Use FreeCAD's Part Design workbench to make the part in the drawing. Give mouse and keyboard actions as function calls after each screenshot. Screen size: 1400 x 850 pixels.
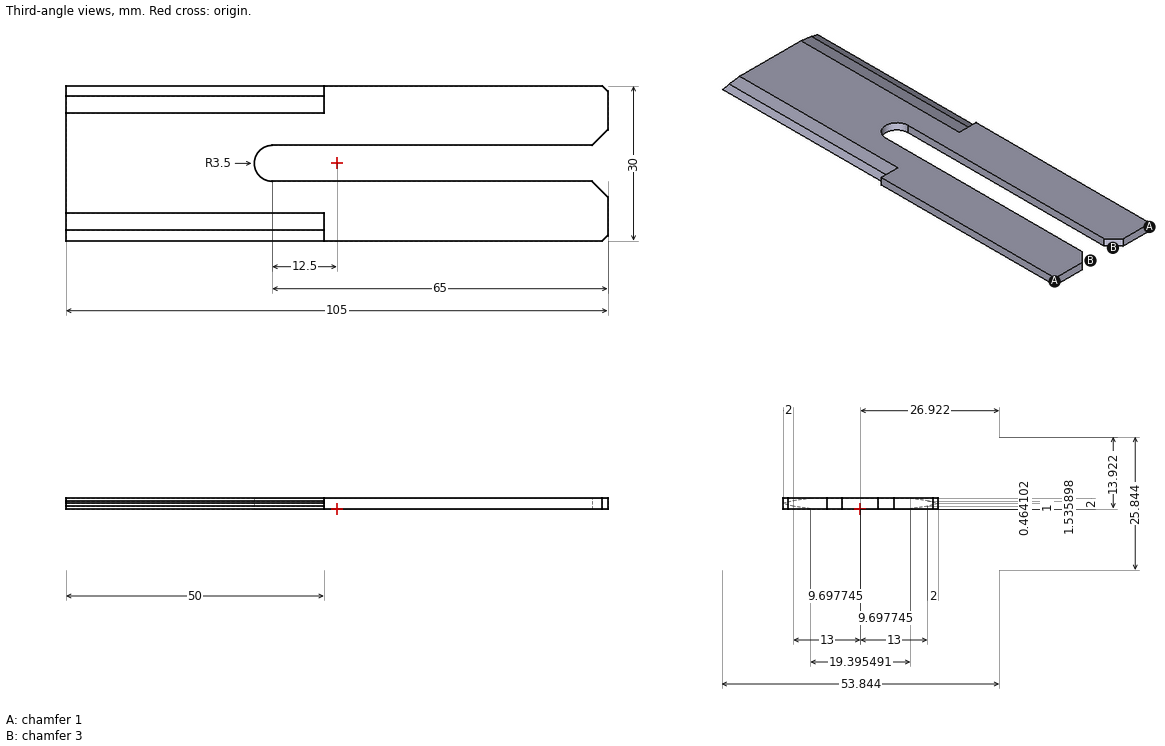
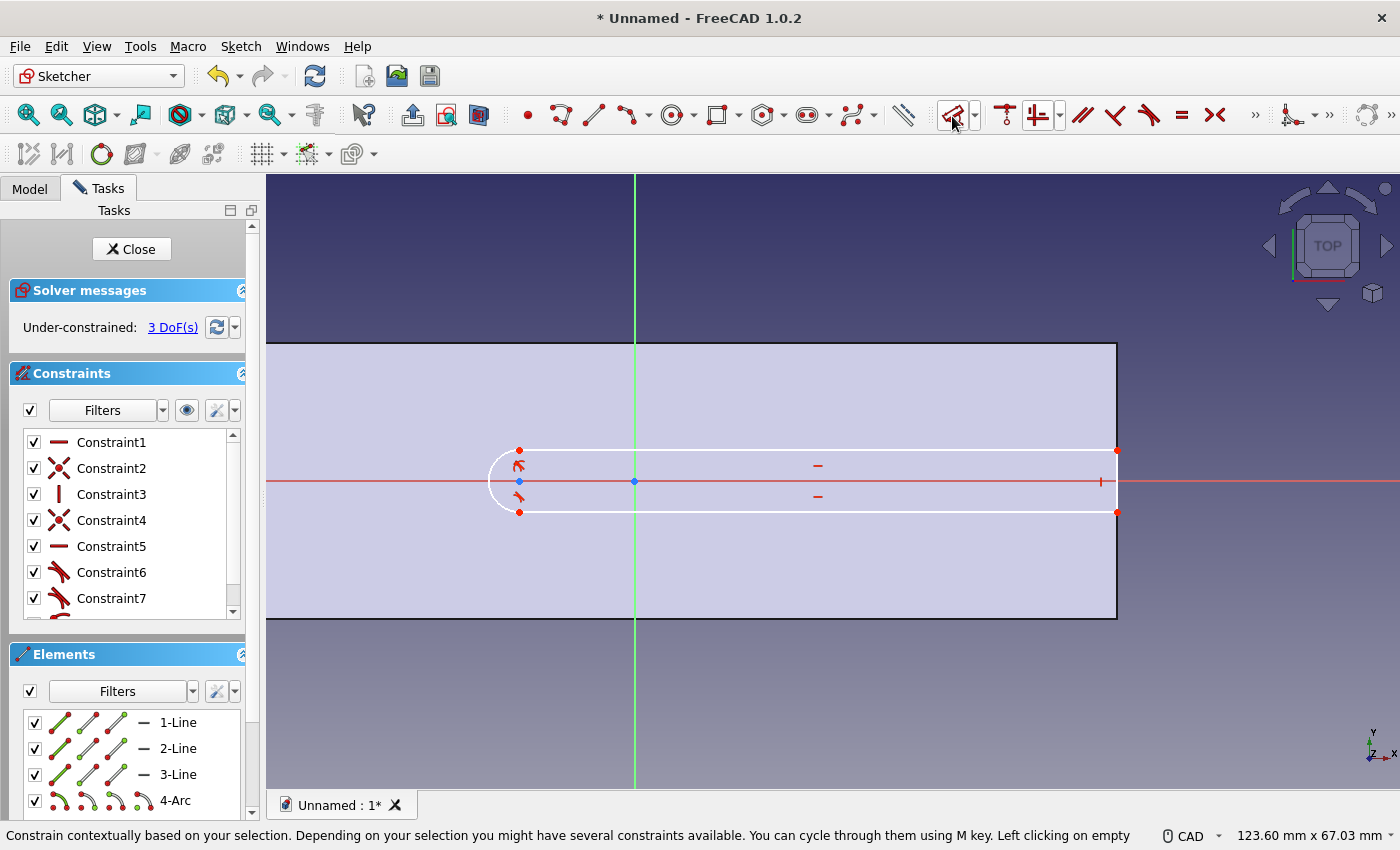
scroll(495, 463, up, 2)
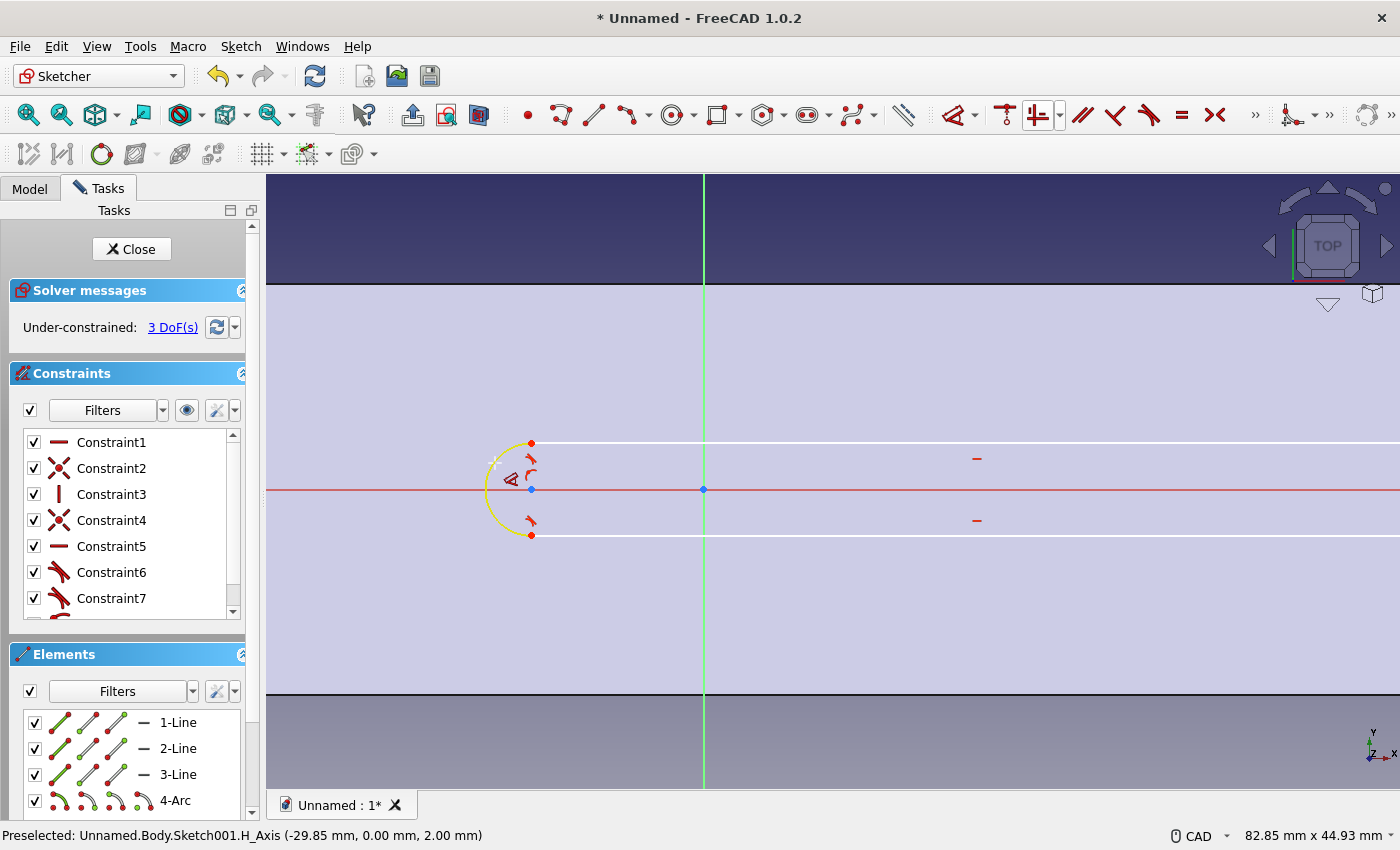
click(494, 462)
click(468, 443)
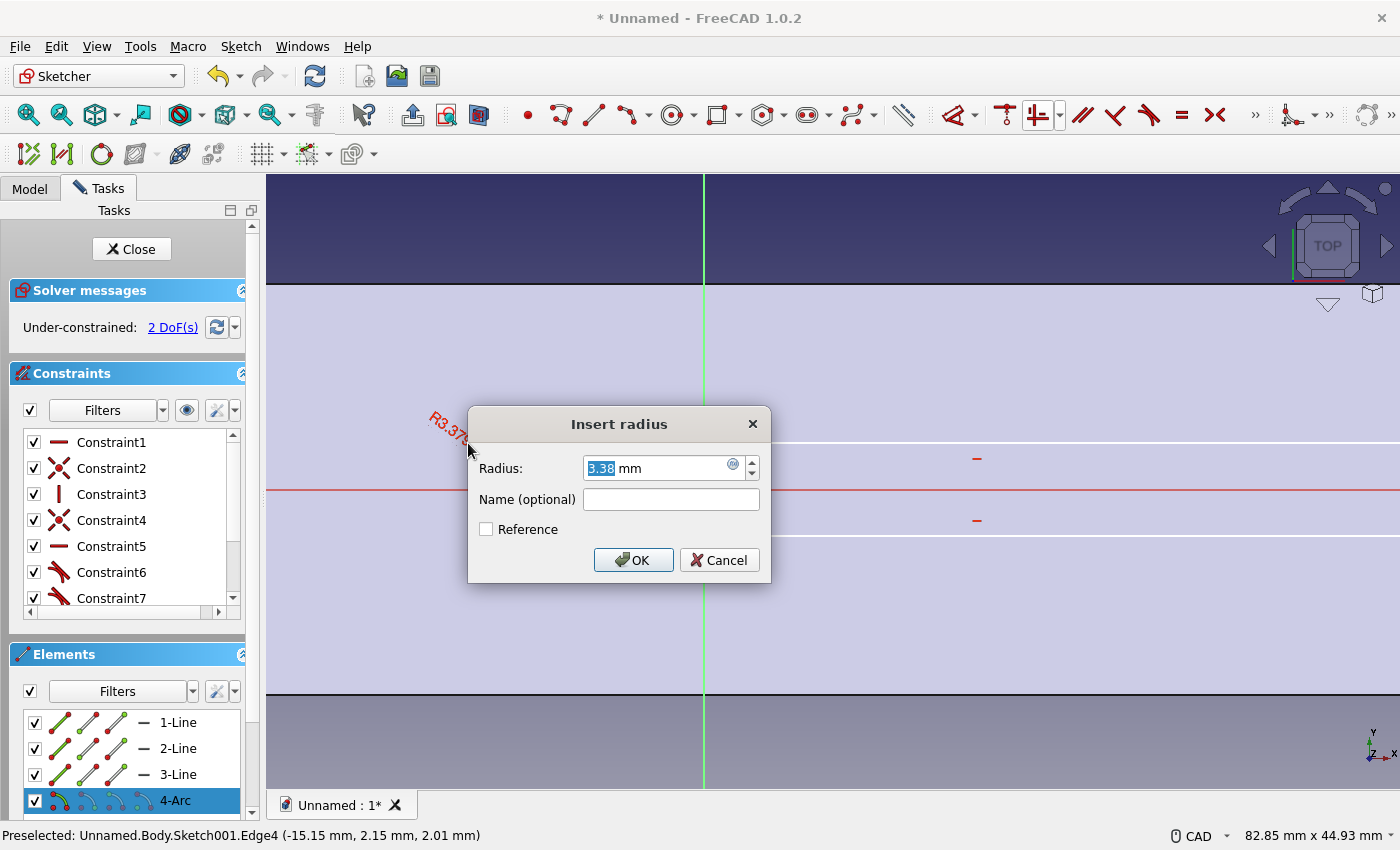
text(3.5)
key(Return)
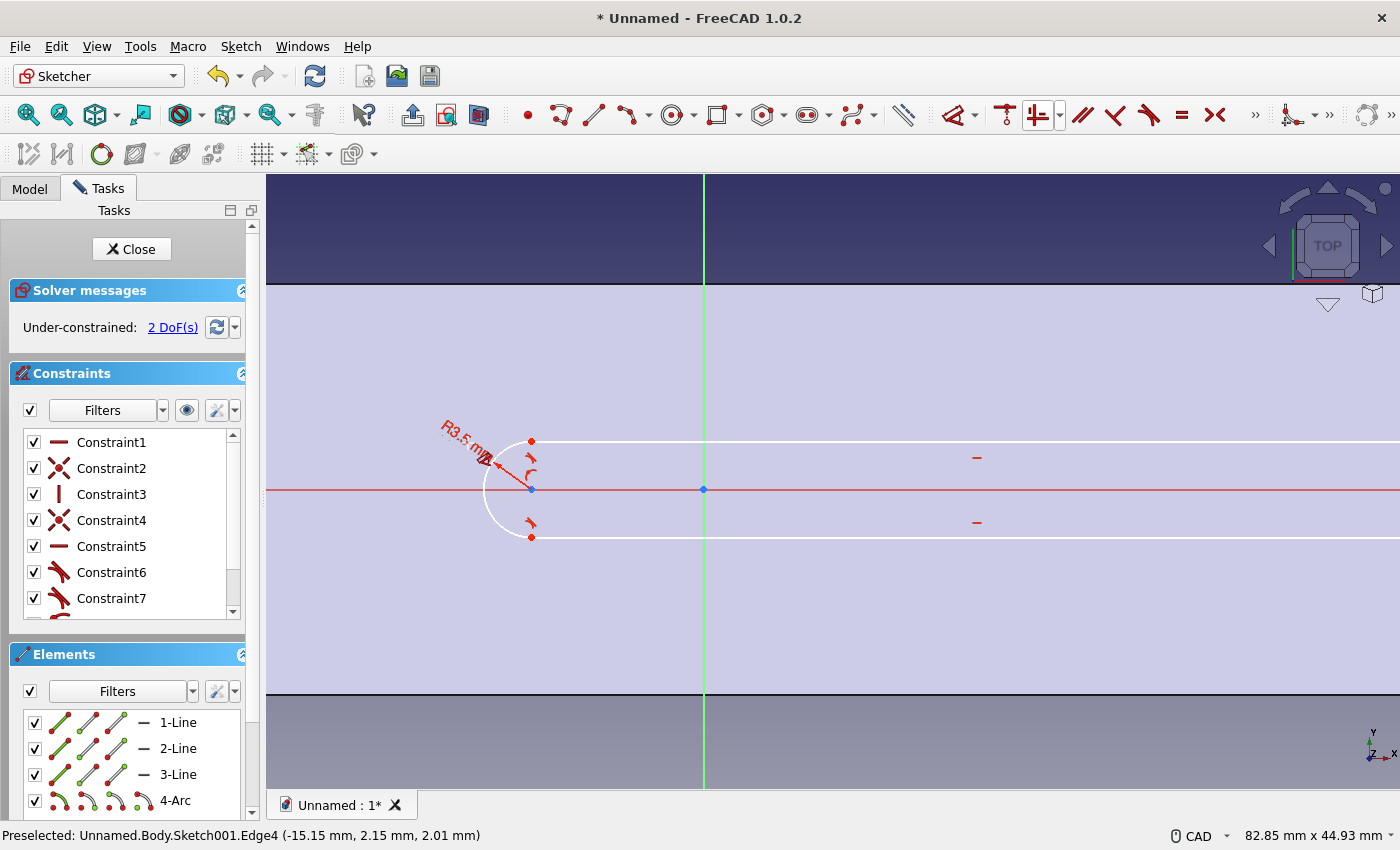
click(799, 538)
click(883, 572)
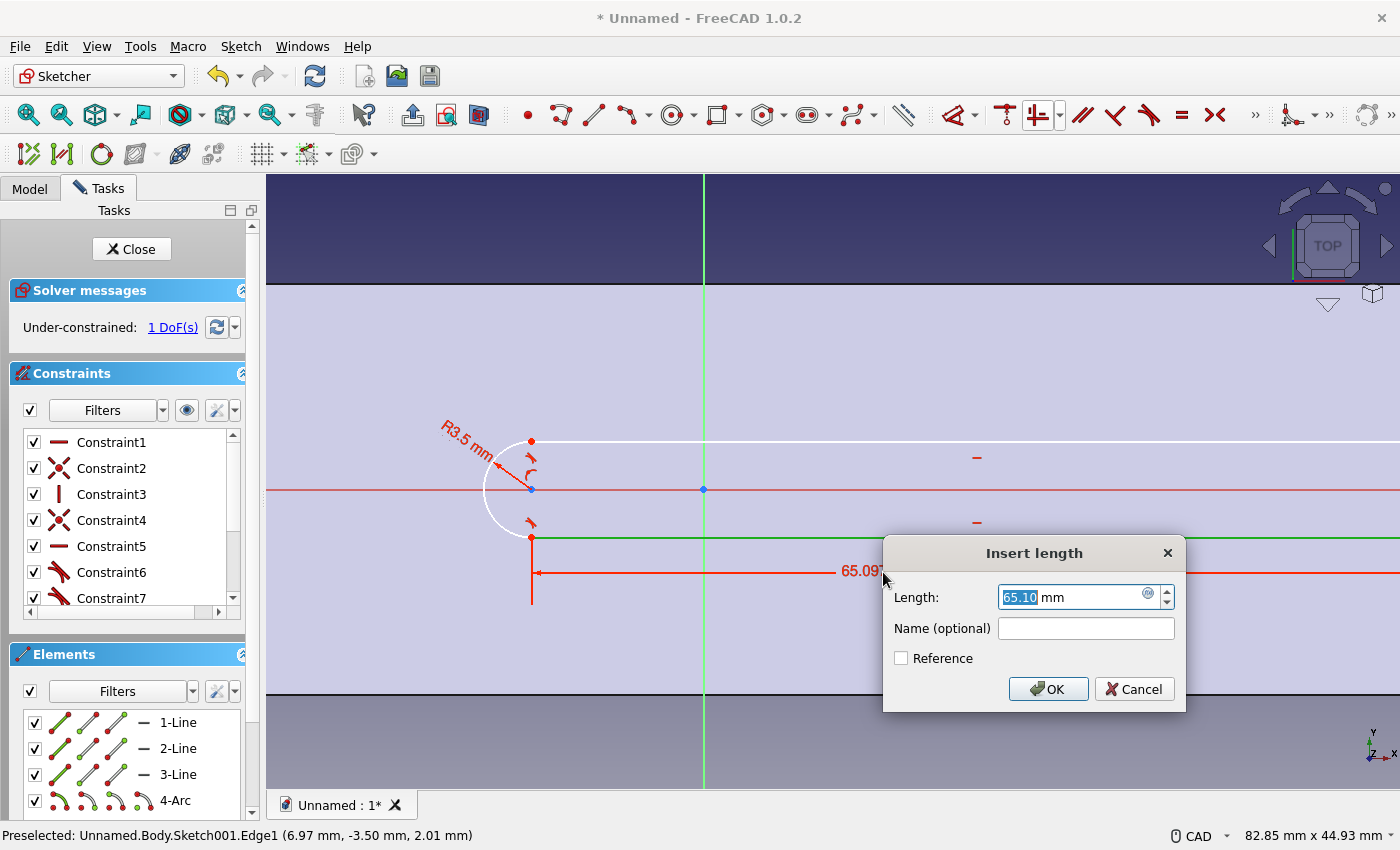
text(65)
key(Return)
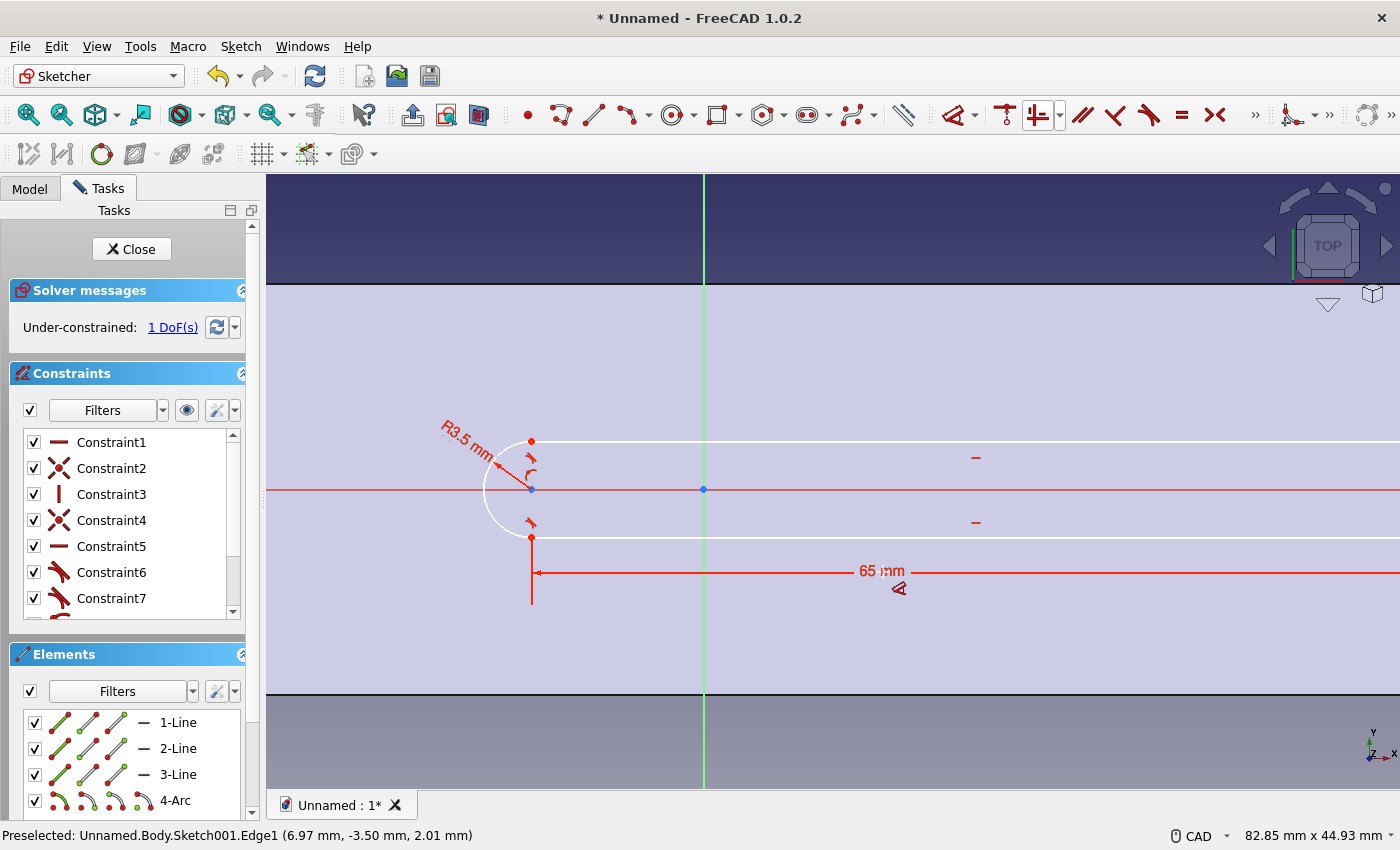
click(532, 538)
click(618, 572)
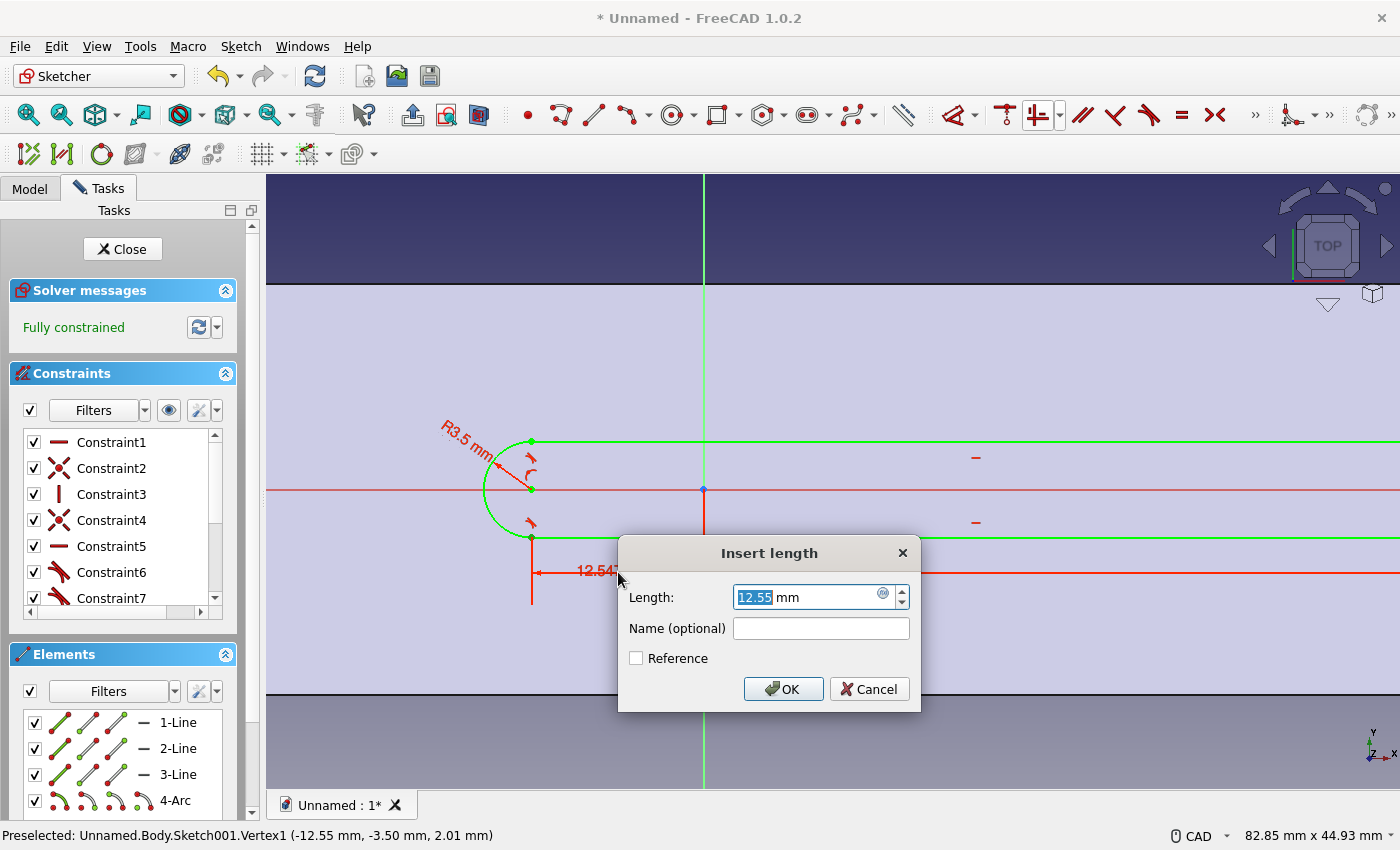
text(12.5)
key(Return)
key(Escape)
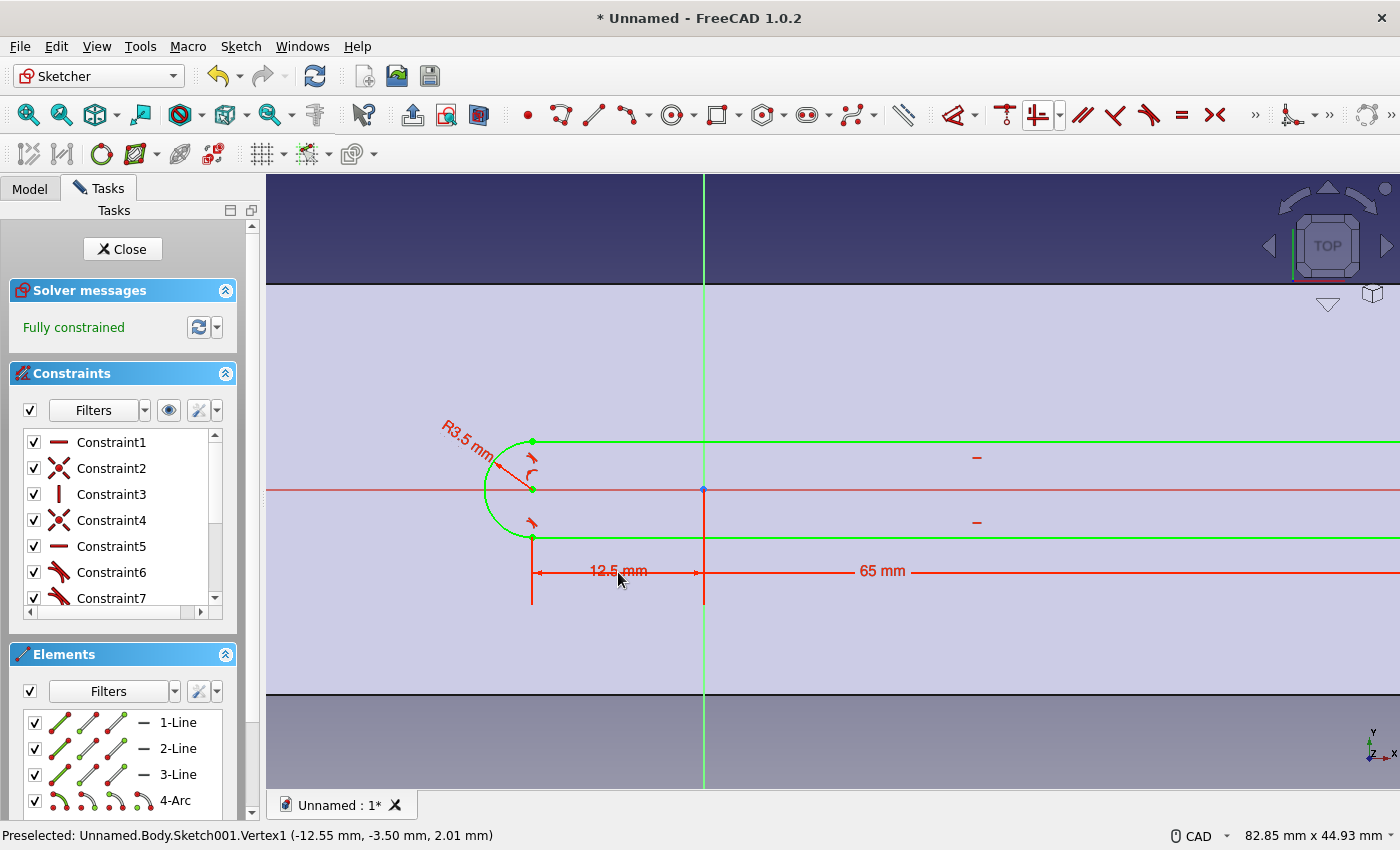
click(123, 249)